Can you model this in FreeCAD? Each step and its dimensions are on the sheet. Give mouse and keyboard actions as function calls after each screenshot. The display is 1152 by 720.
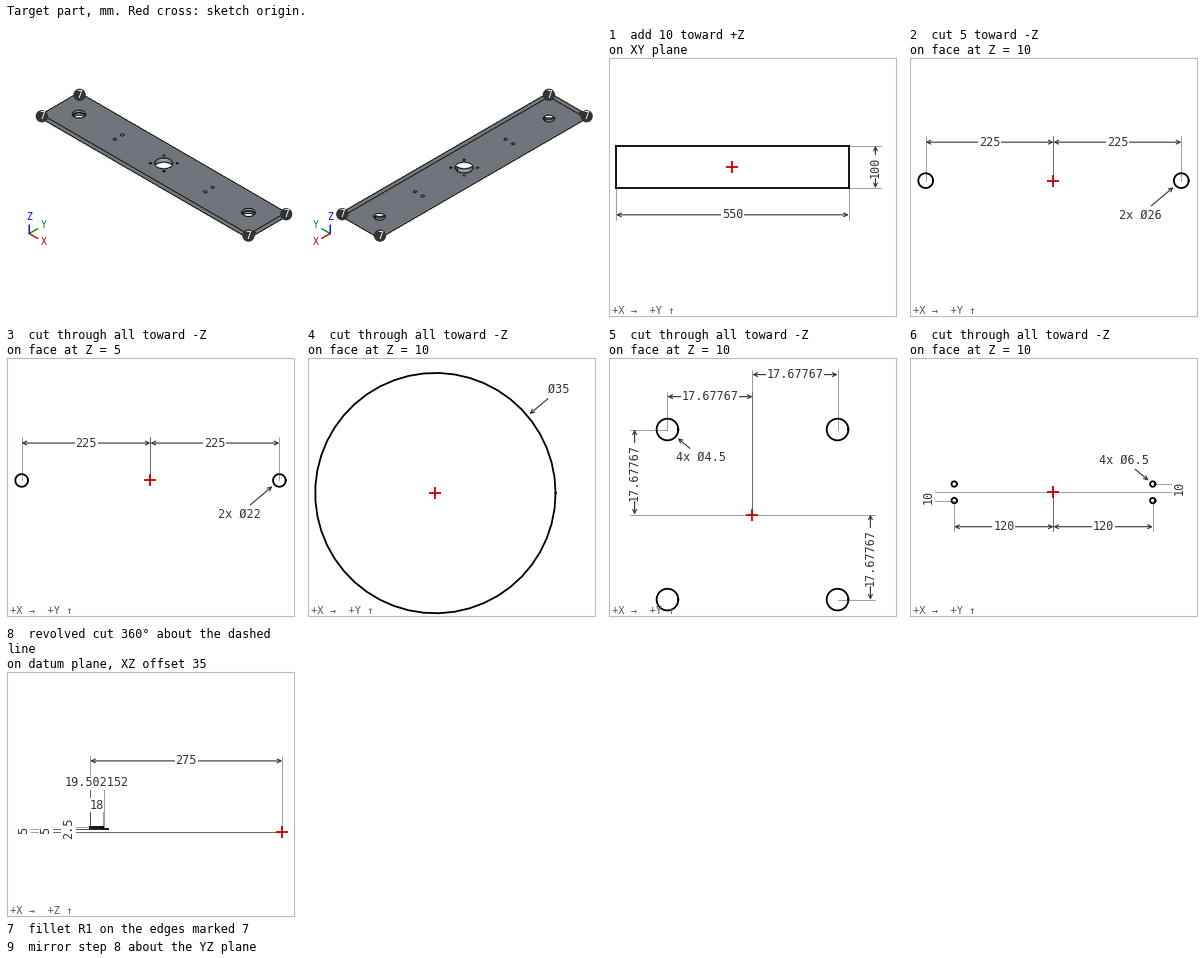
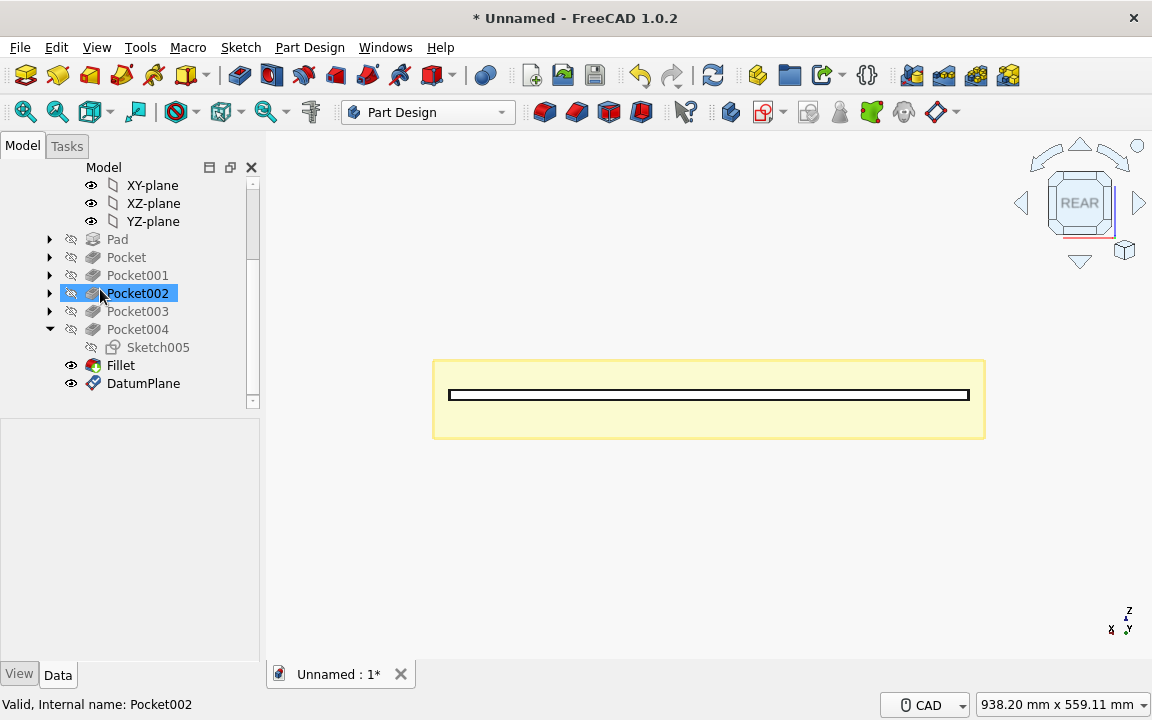
click(116, 383)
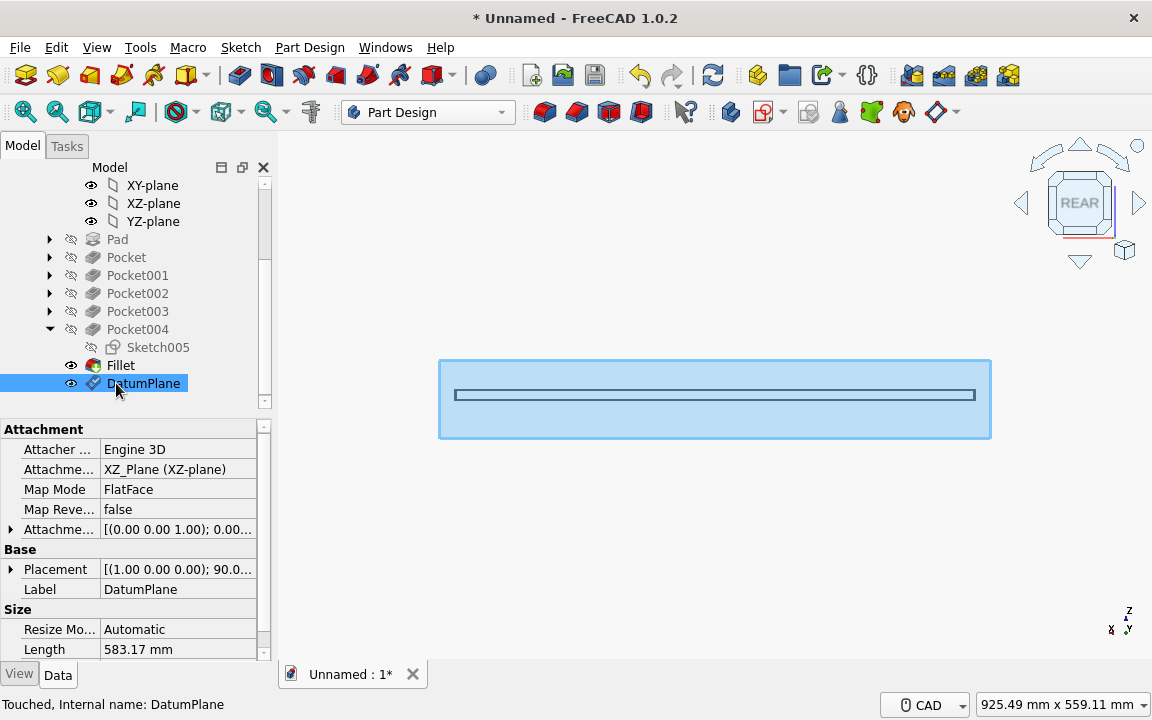
click(764, 112)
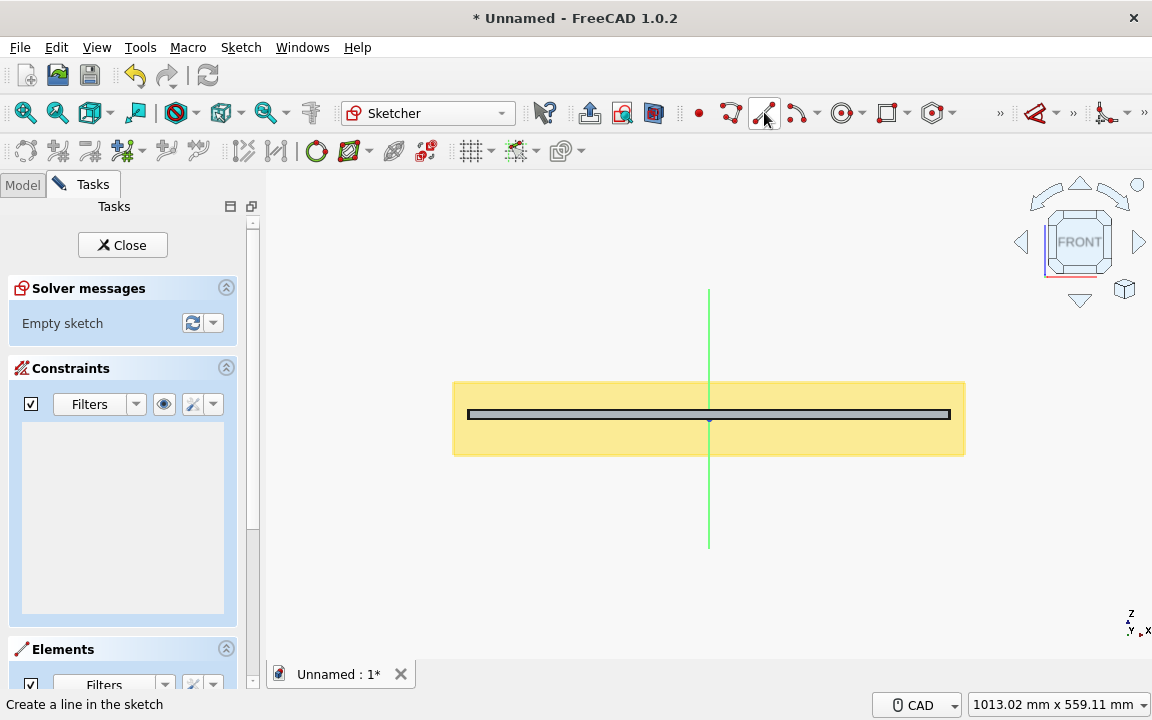
click(654, 114)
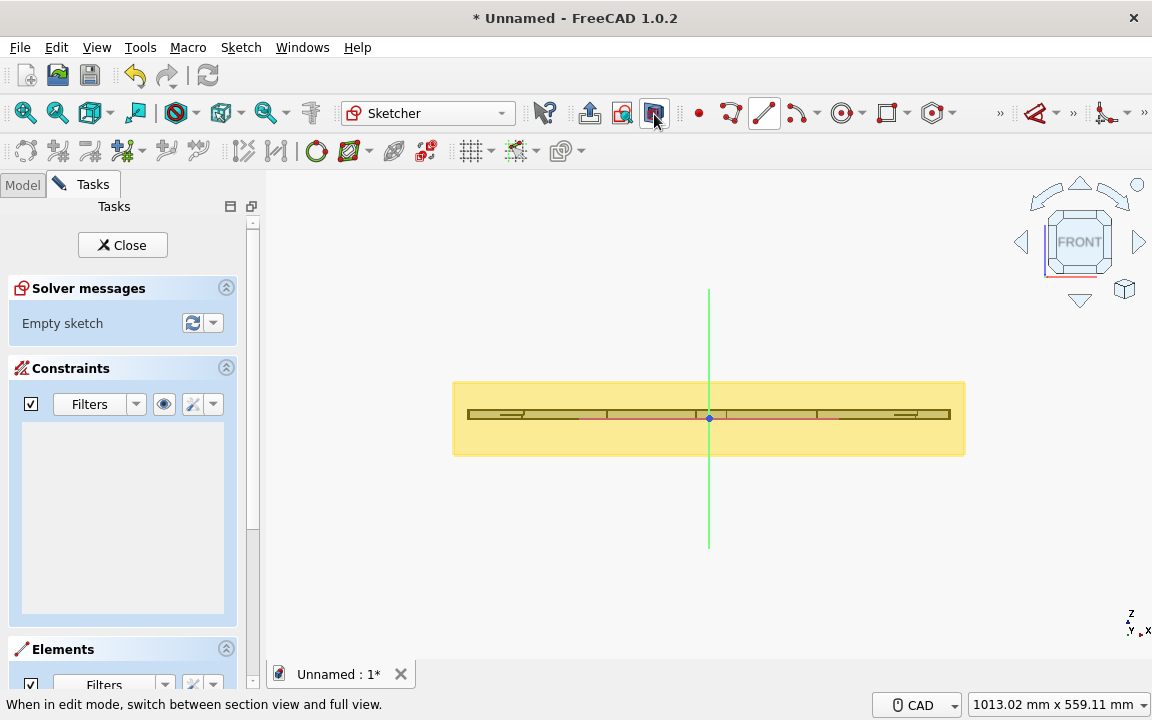
scroll(472, 413, up, 15)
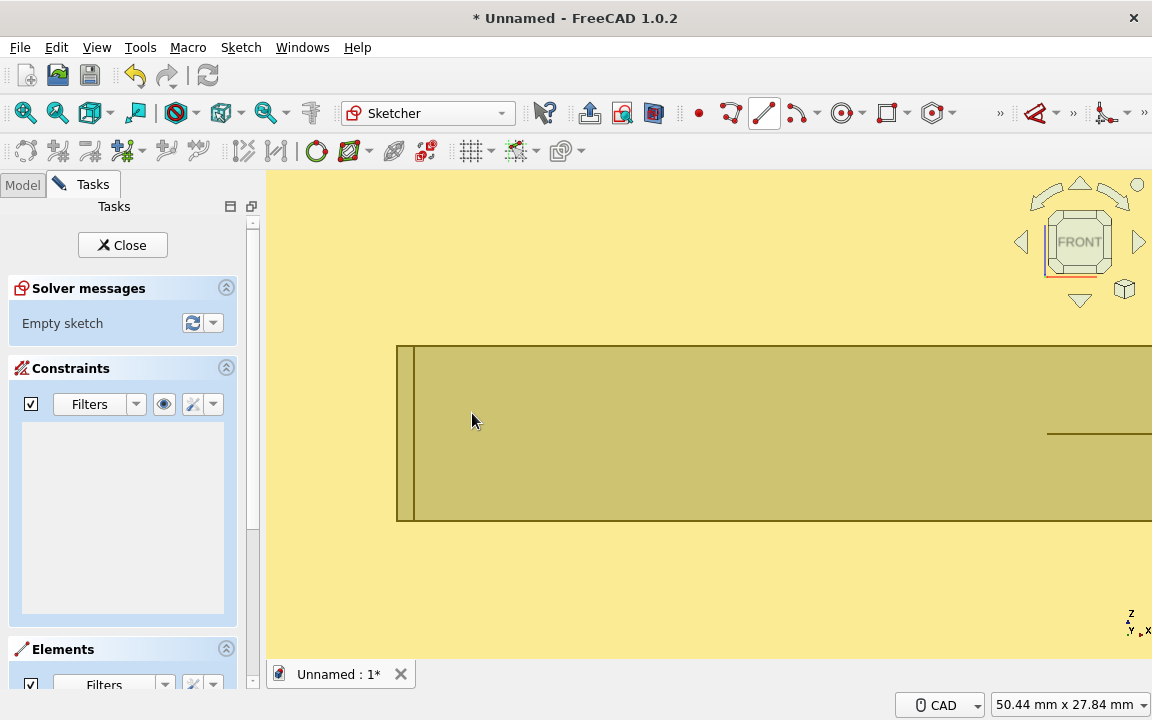
click(732, 114)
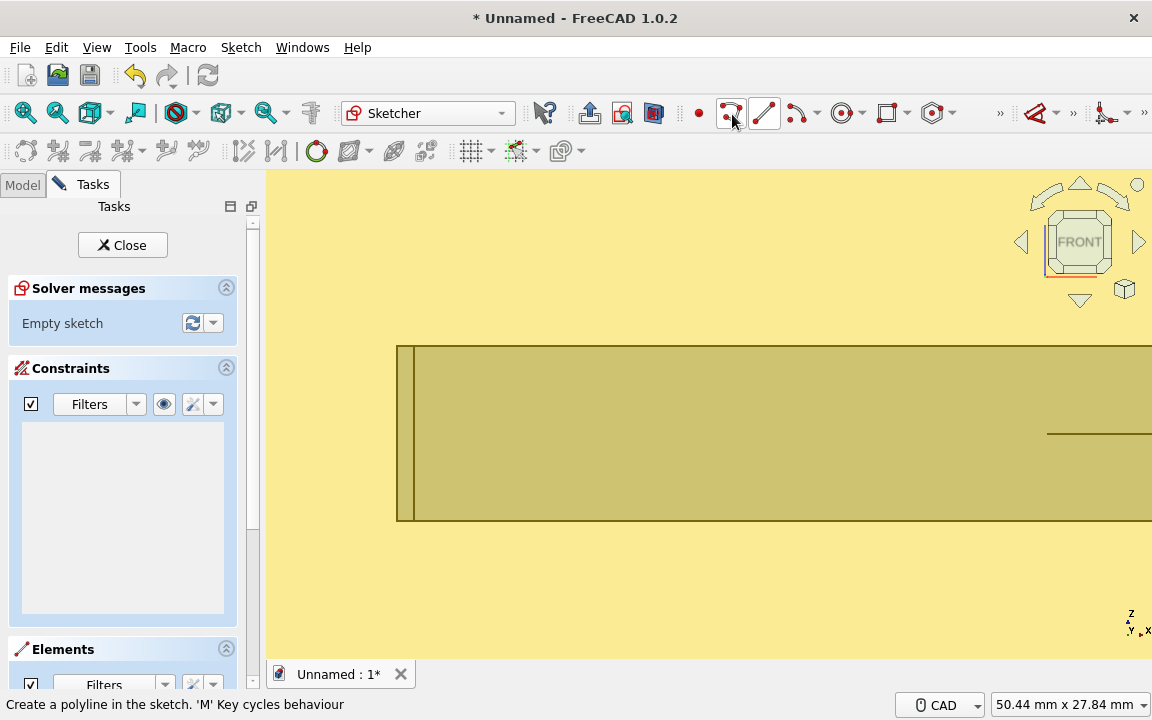
click(739, 434)
click(397, 434)
click(397, 390)
click(713, 390)
click(739, 435)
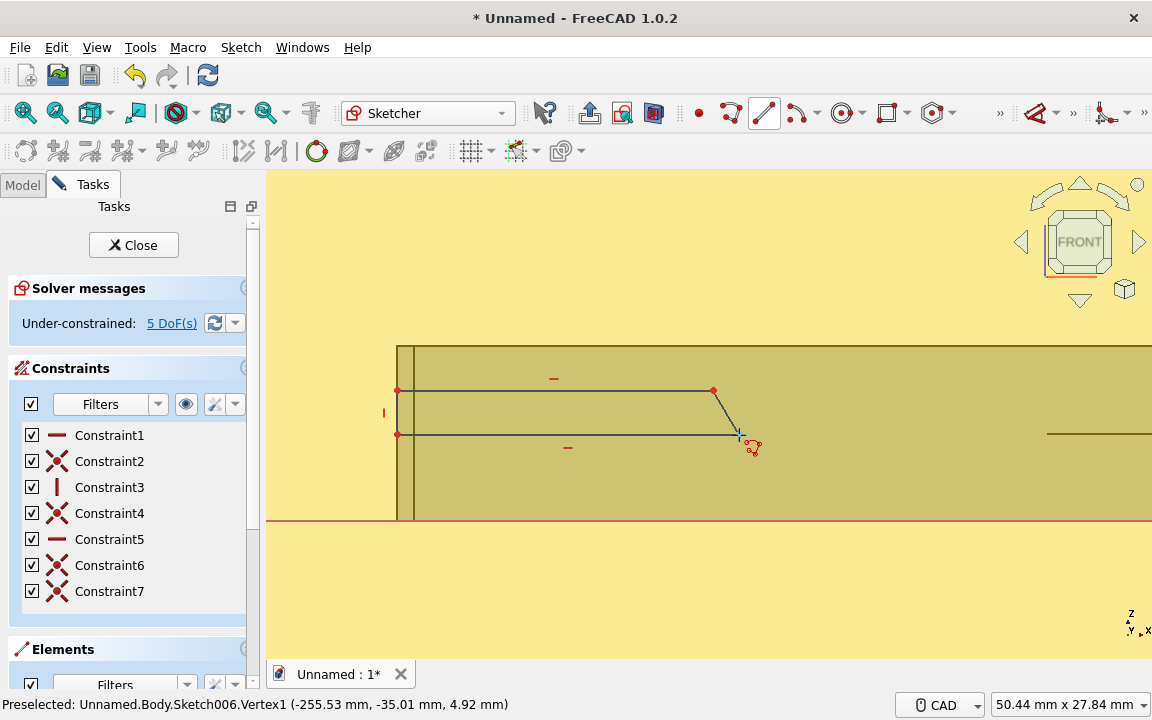
click(764, 114)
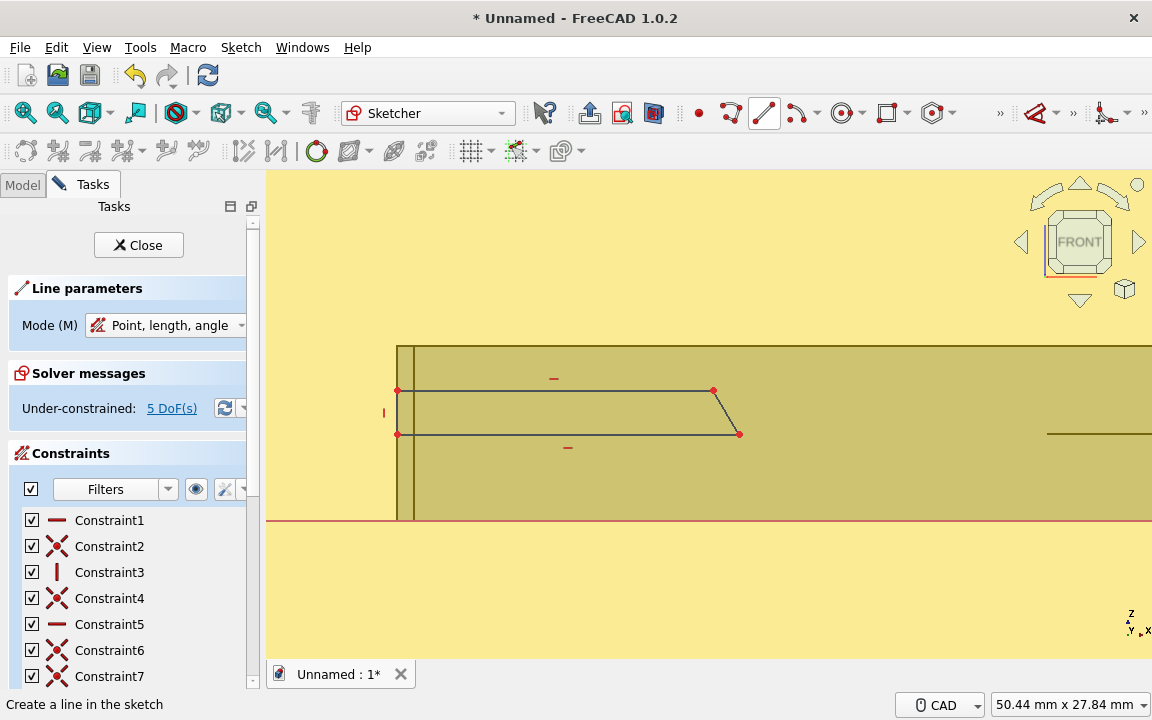
click(774, 434)
click(877, 434)
key(Escape)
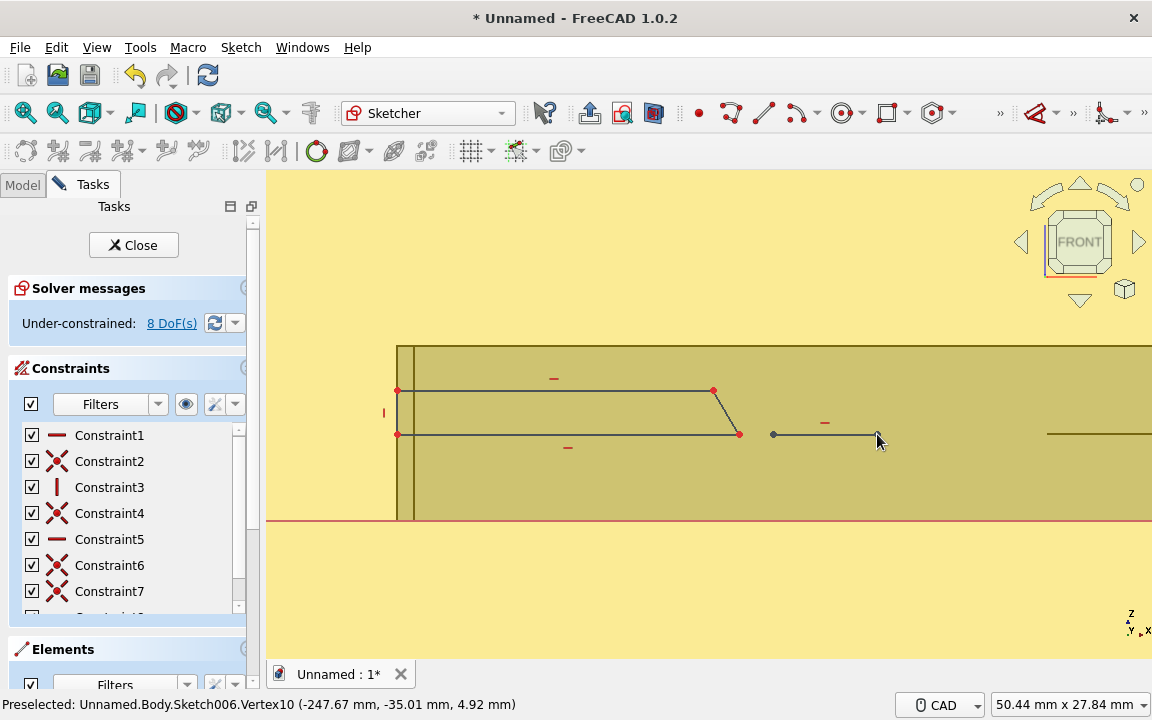
click(805, 435)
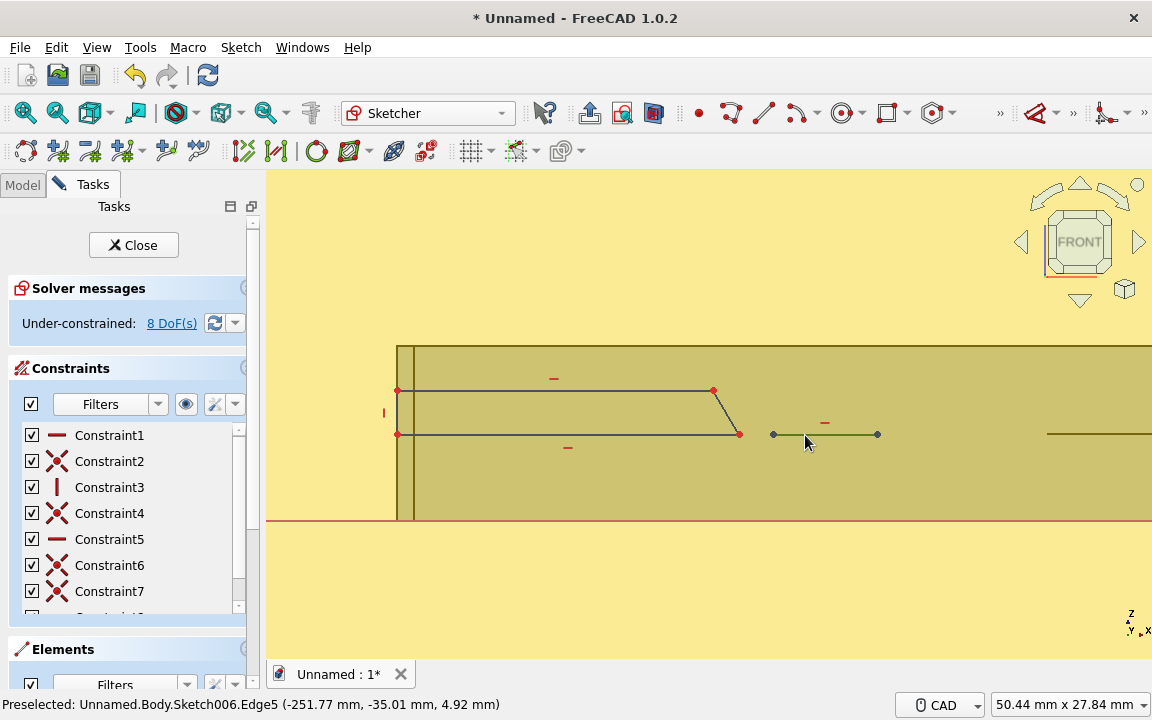
key(g)
key(n)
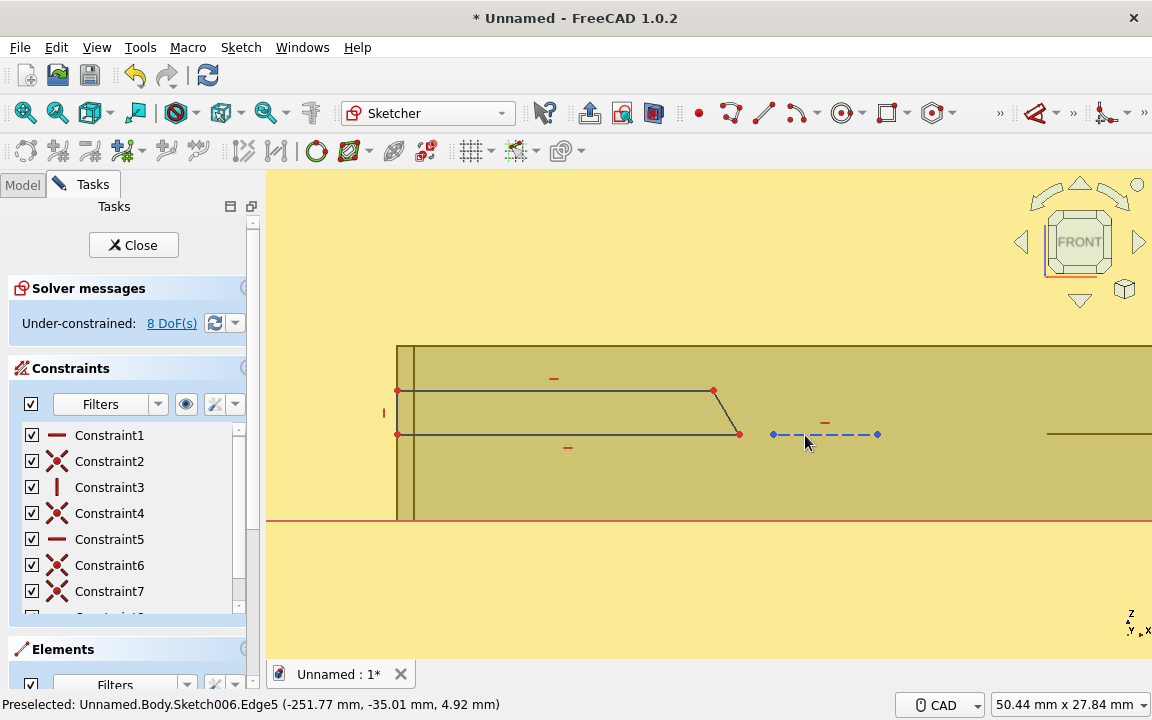
click(1036, 114)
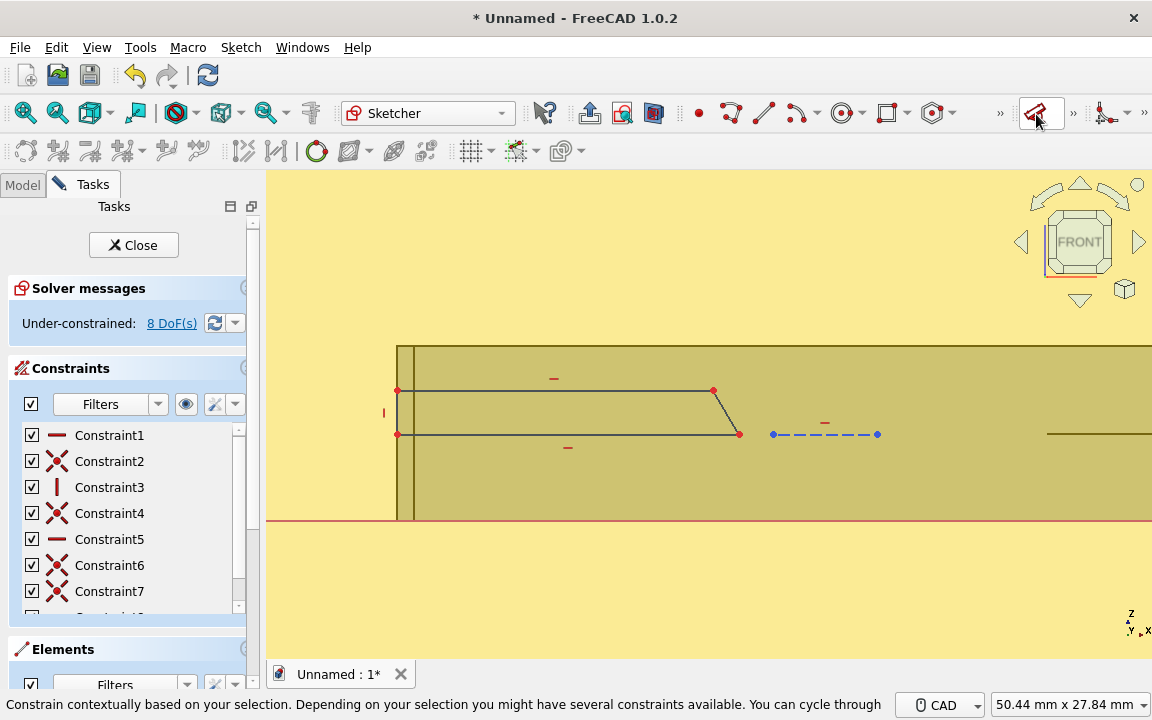
click(492, 391)
click(555, 357)